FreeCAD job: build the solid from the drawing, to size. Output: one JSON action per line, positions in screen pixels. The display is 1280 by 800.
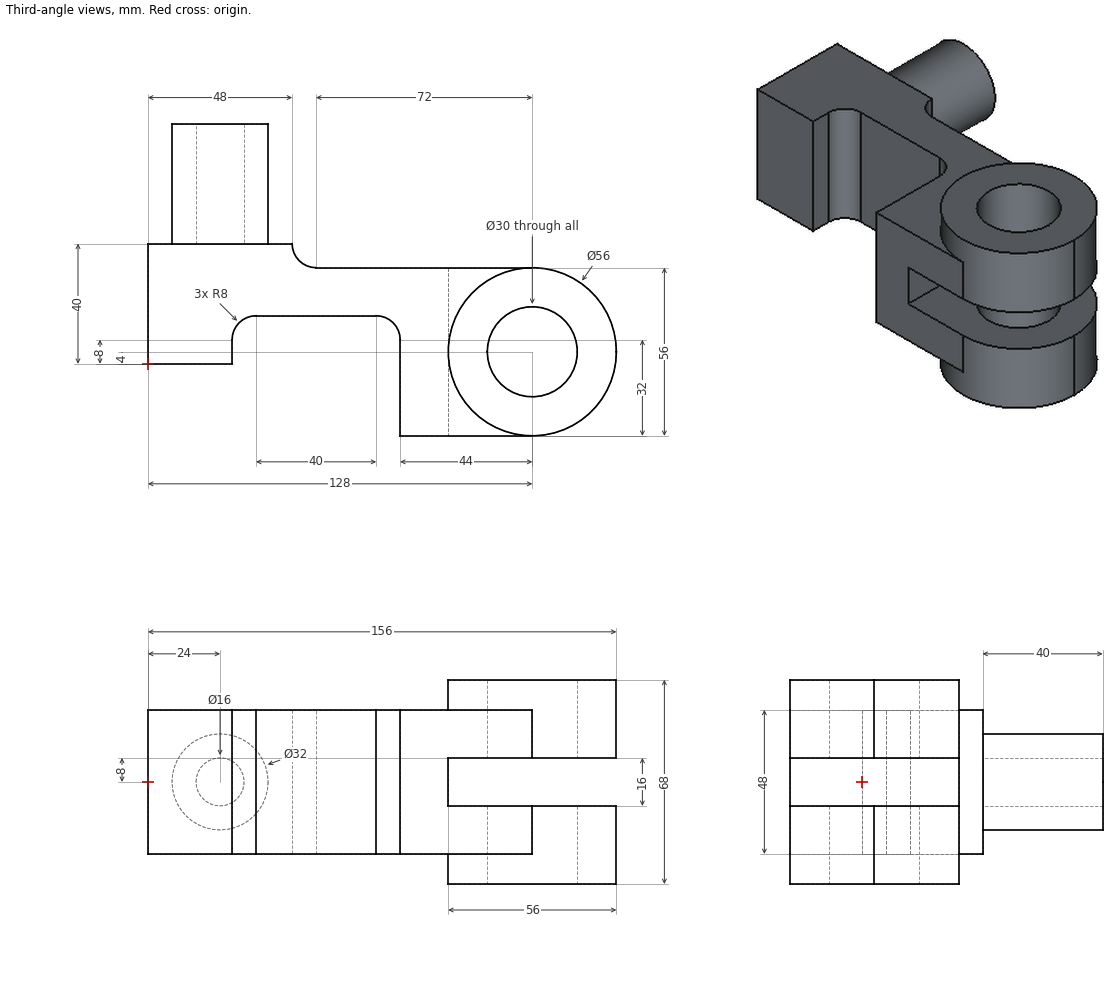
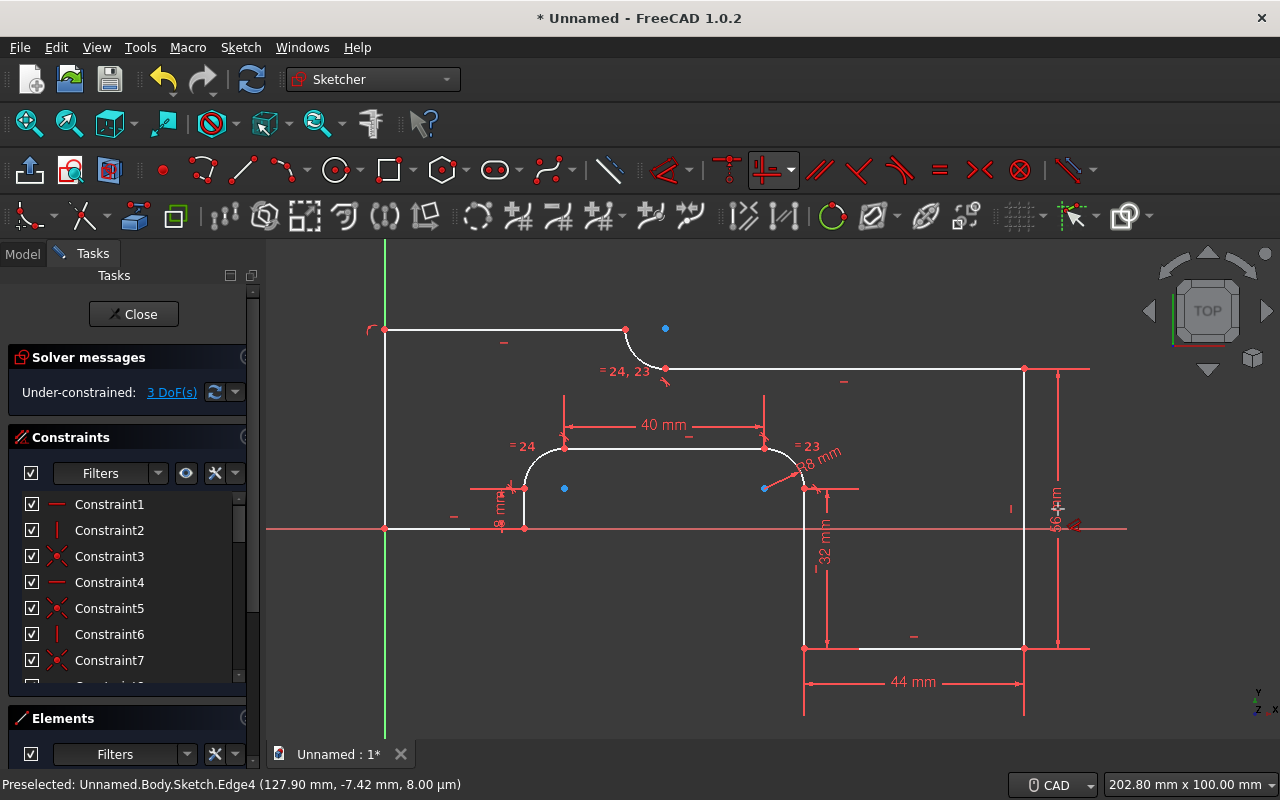
{"action": "left_click", "coordinate": [917, 369]}
{"action": "left_click", "coordinate": [845, 335]}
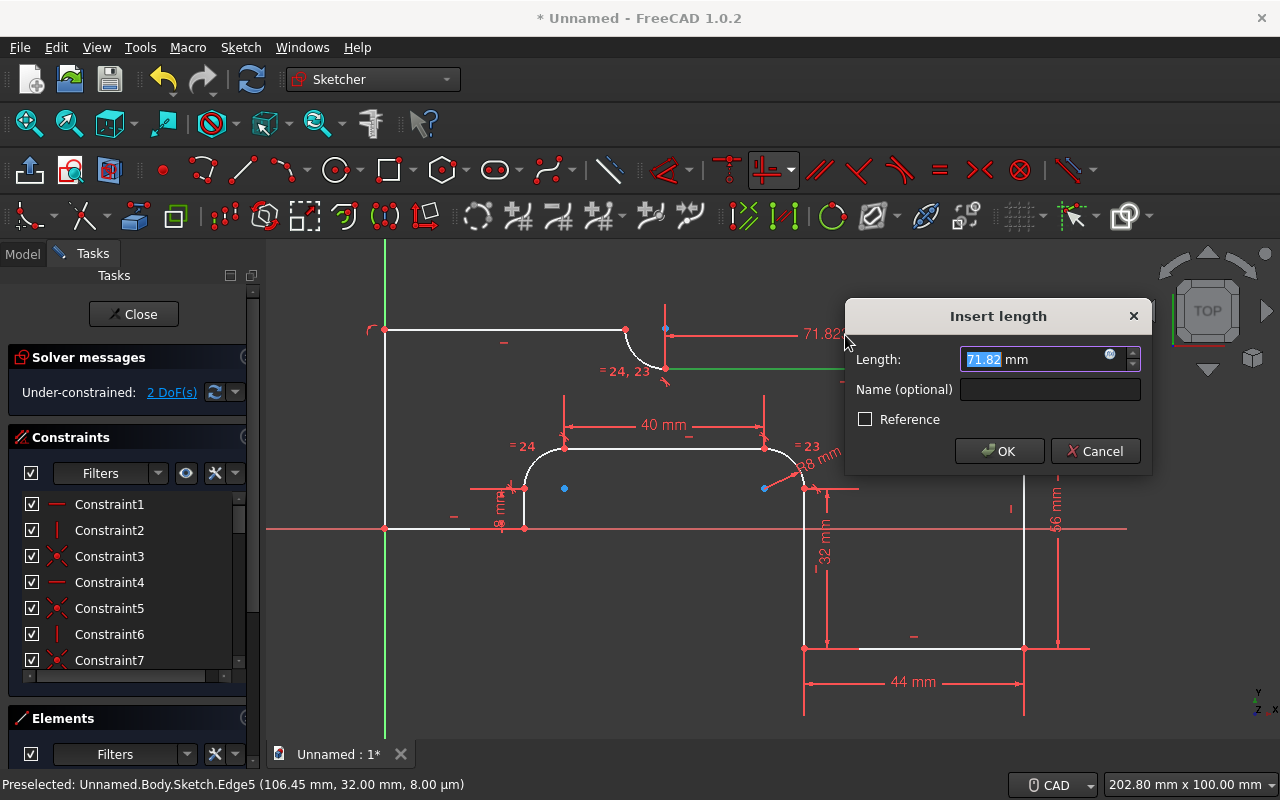
{"action": "type", "text": "72"}
{"action": "key", "text": "Return"}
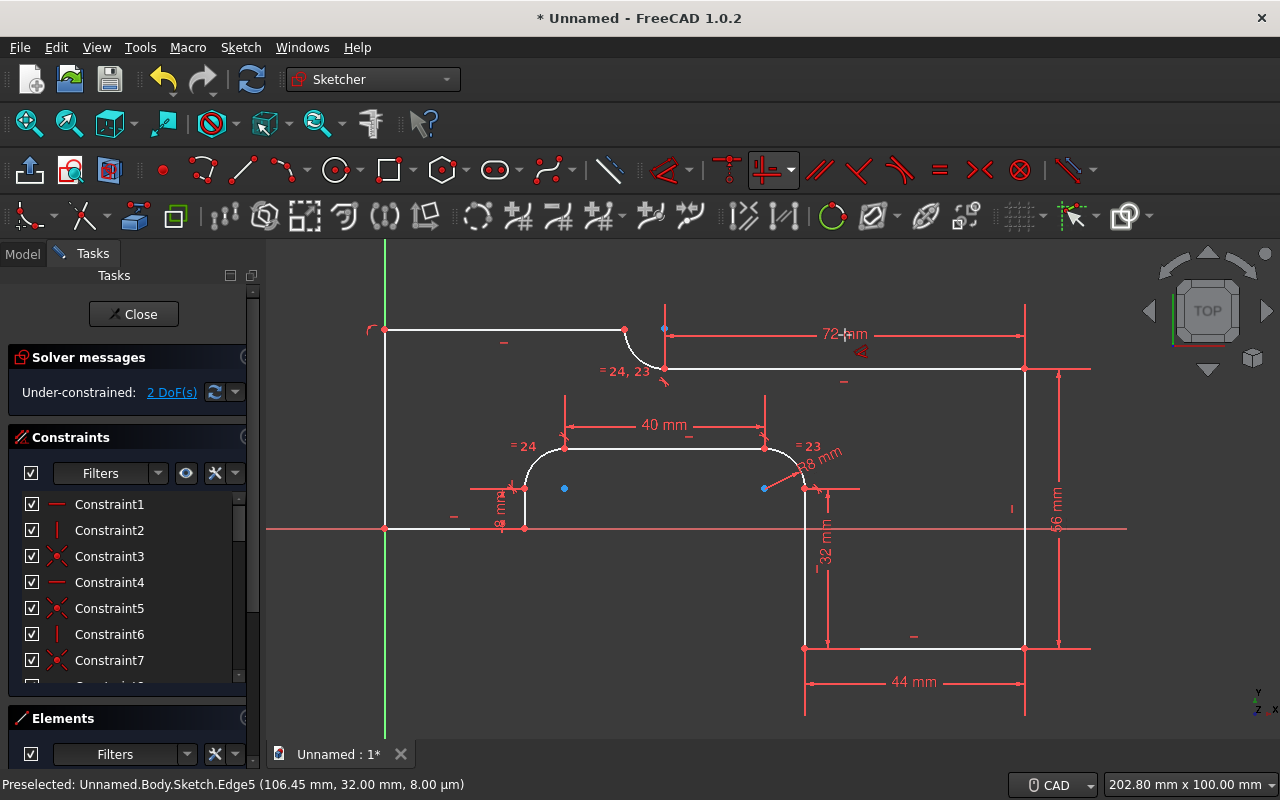
{"action": "left_click", "coordinate": [553, 330]}
{"action": "left_click", "coordinate": [505, 296]}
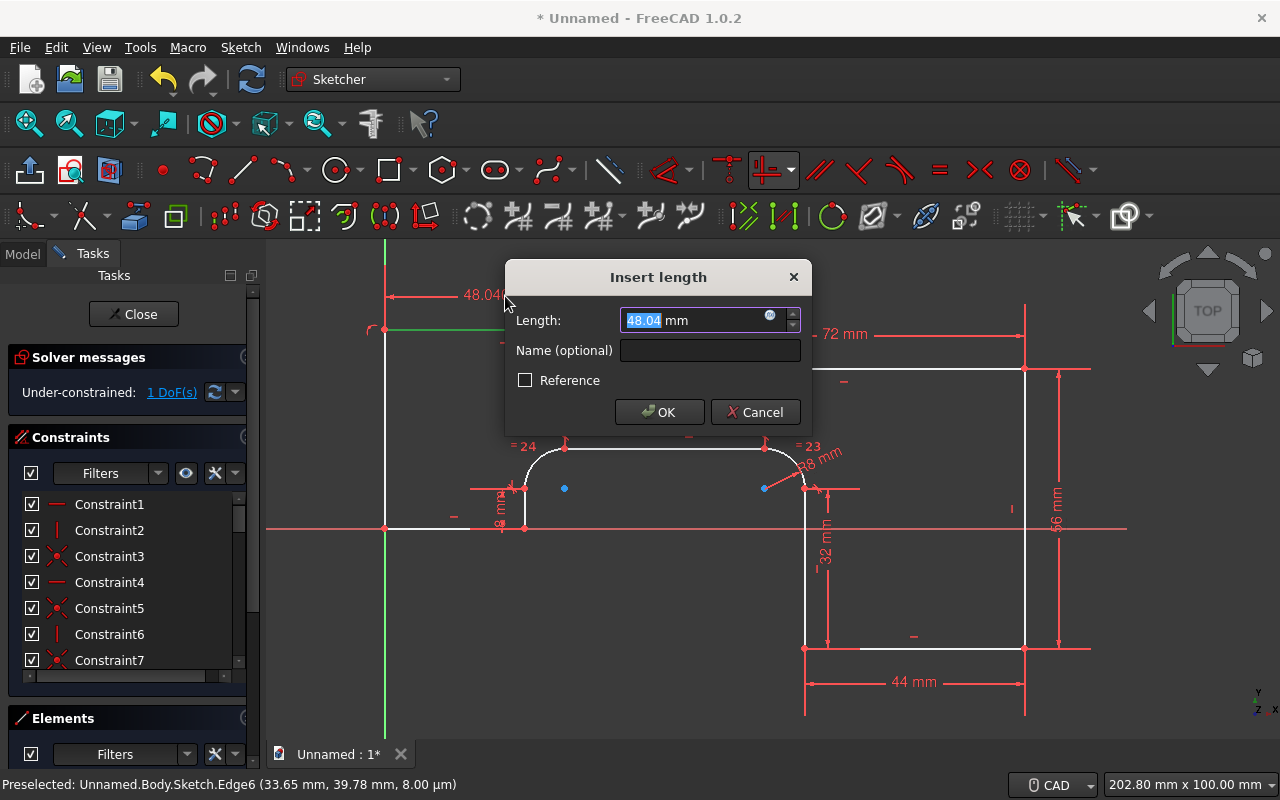
{"action": "type", "text": "48"}
{"action": "key", "text": "Return"}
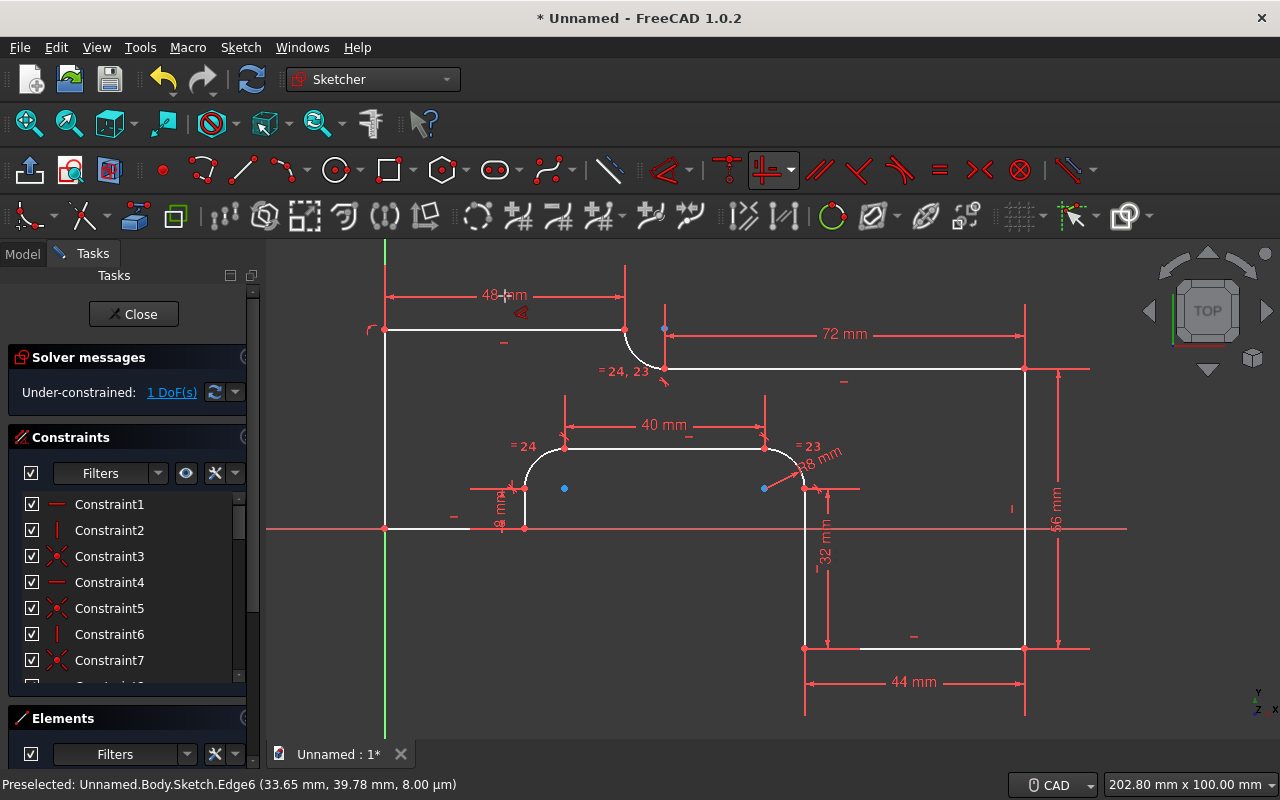
{"action": "left_click", "coordinate": [385, 390]}
{"action": "left_click", "coordinate": [351, 429]}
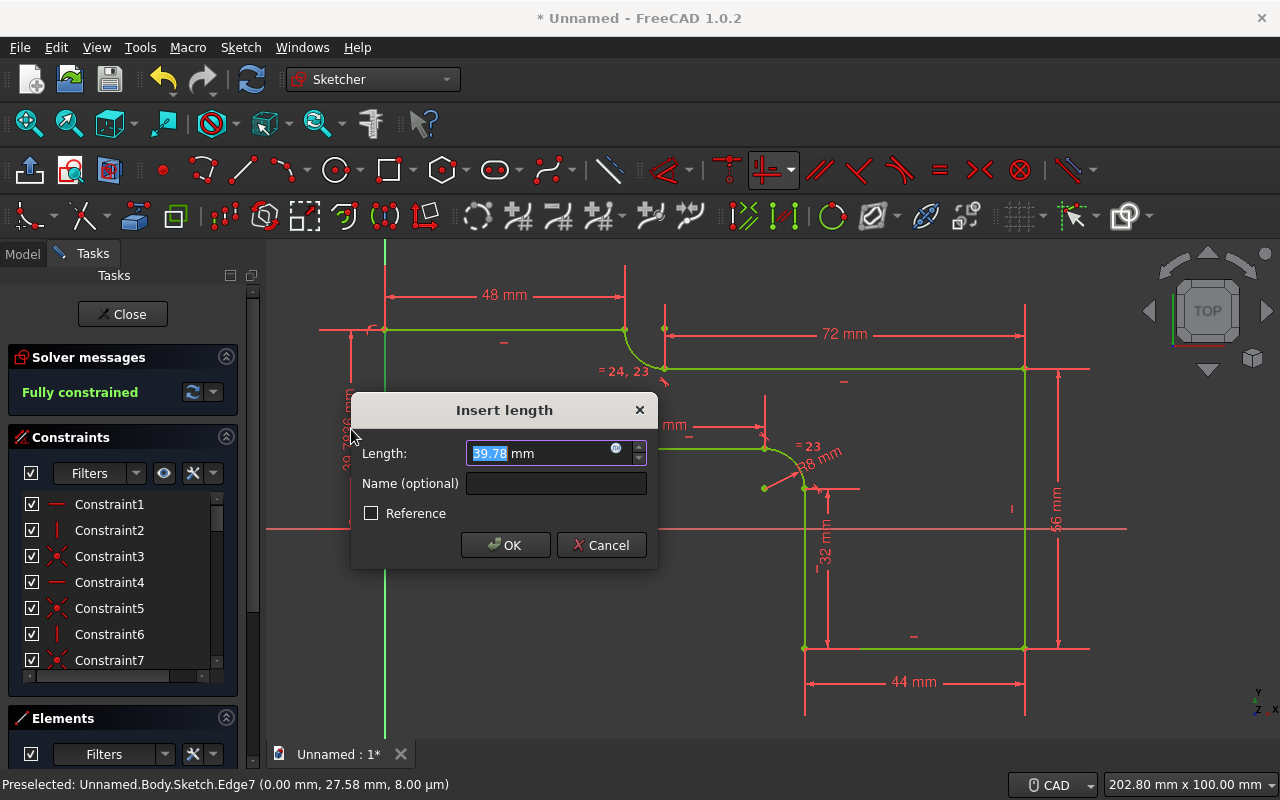
{"action": "type", "text": "40"}
{"action": "key", "text": "Return"}
{"action": "key", "text": "Escape"}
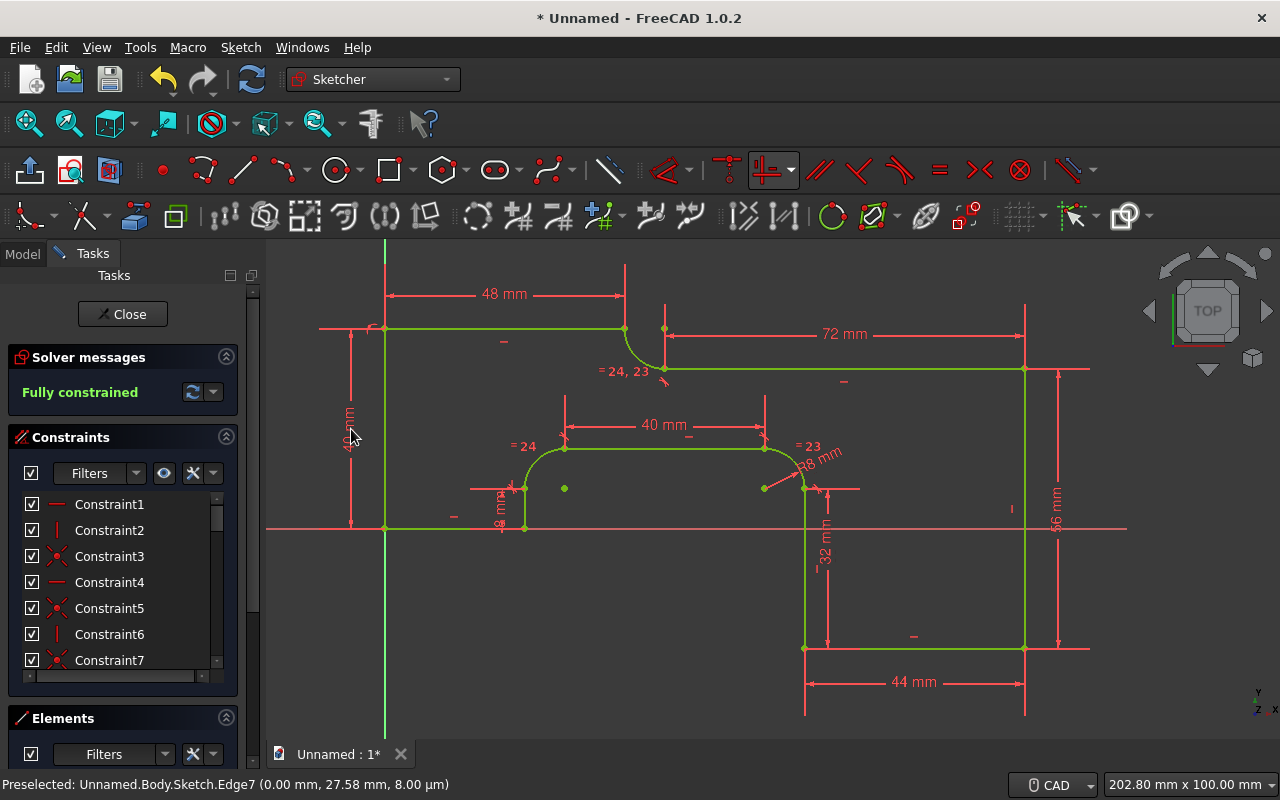
{"action": "left_click", "coordinate": [123, 314]}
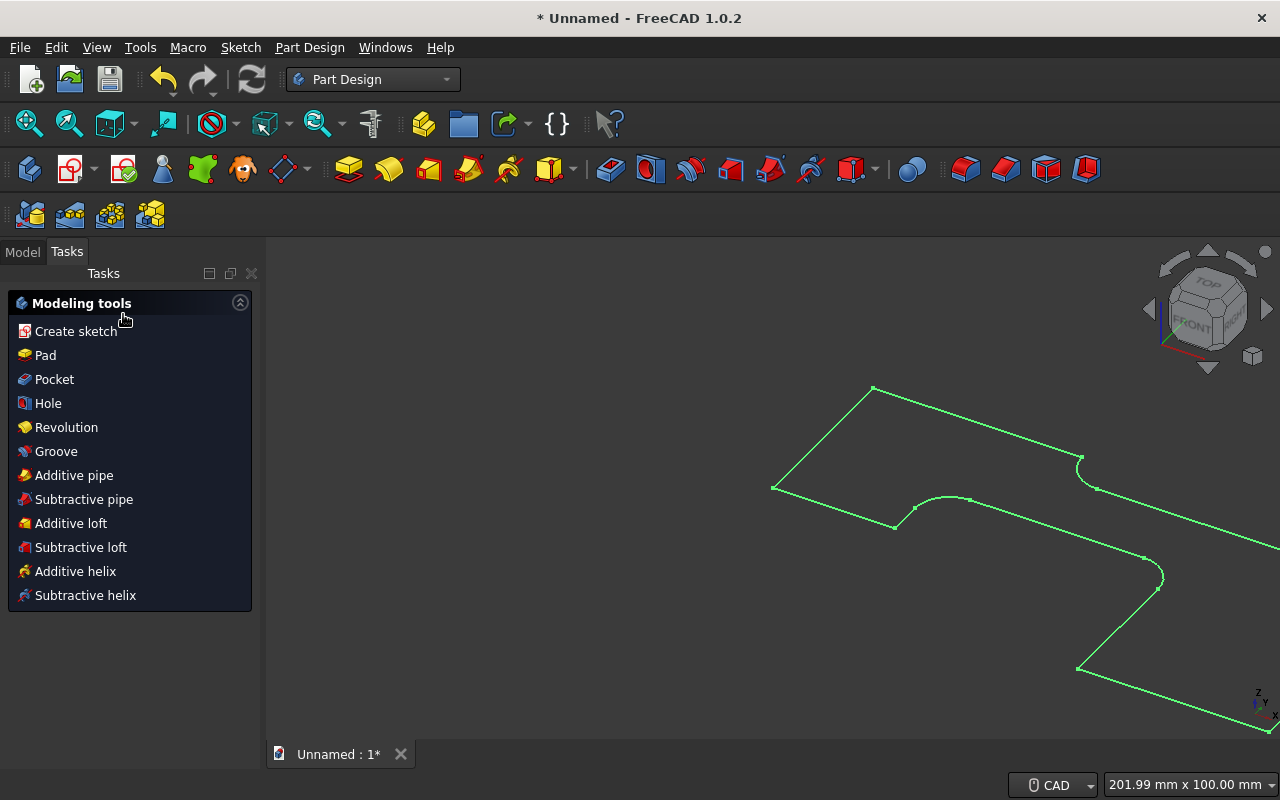
{"action": "left_click", "coordinate": [350, 170]}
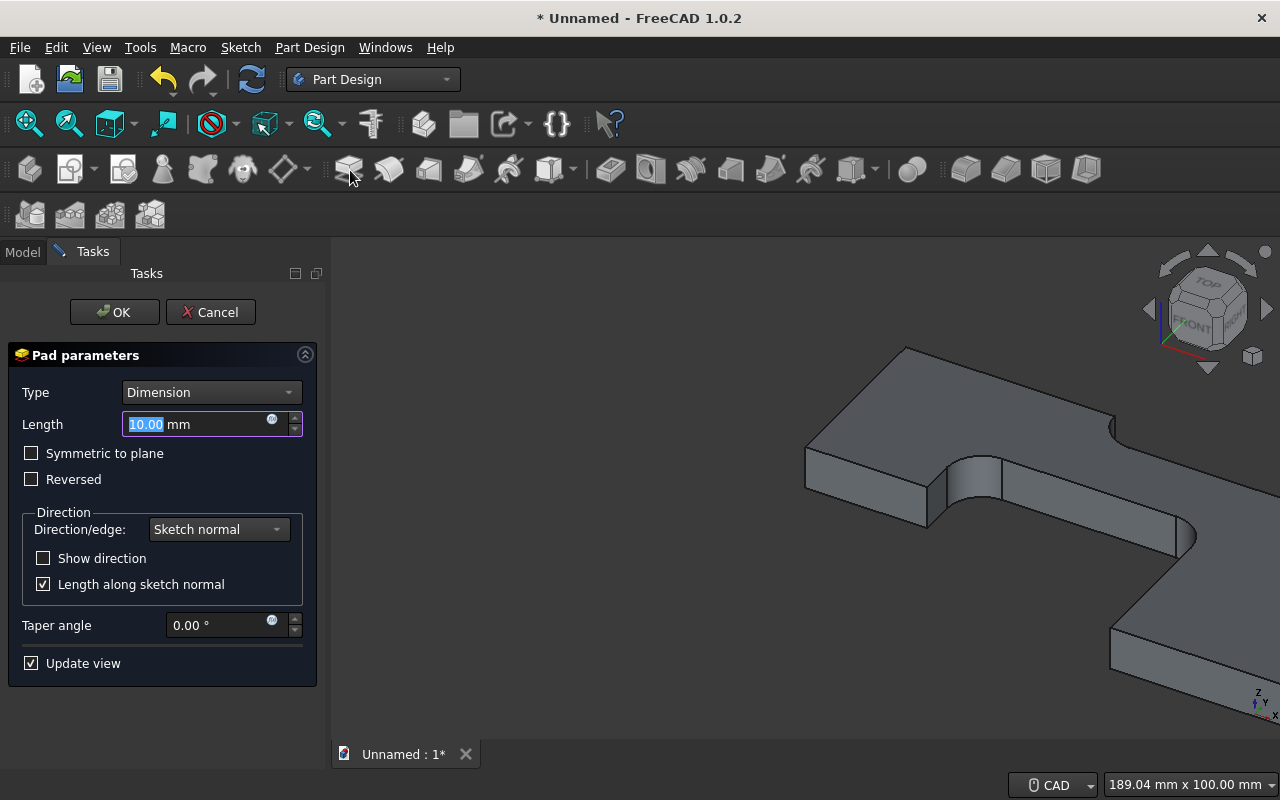
{"action": "type", "text": "48"}
{"action": "key", "text": "Tab"}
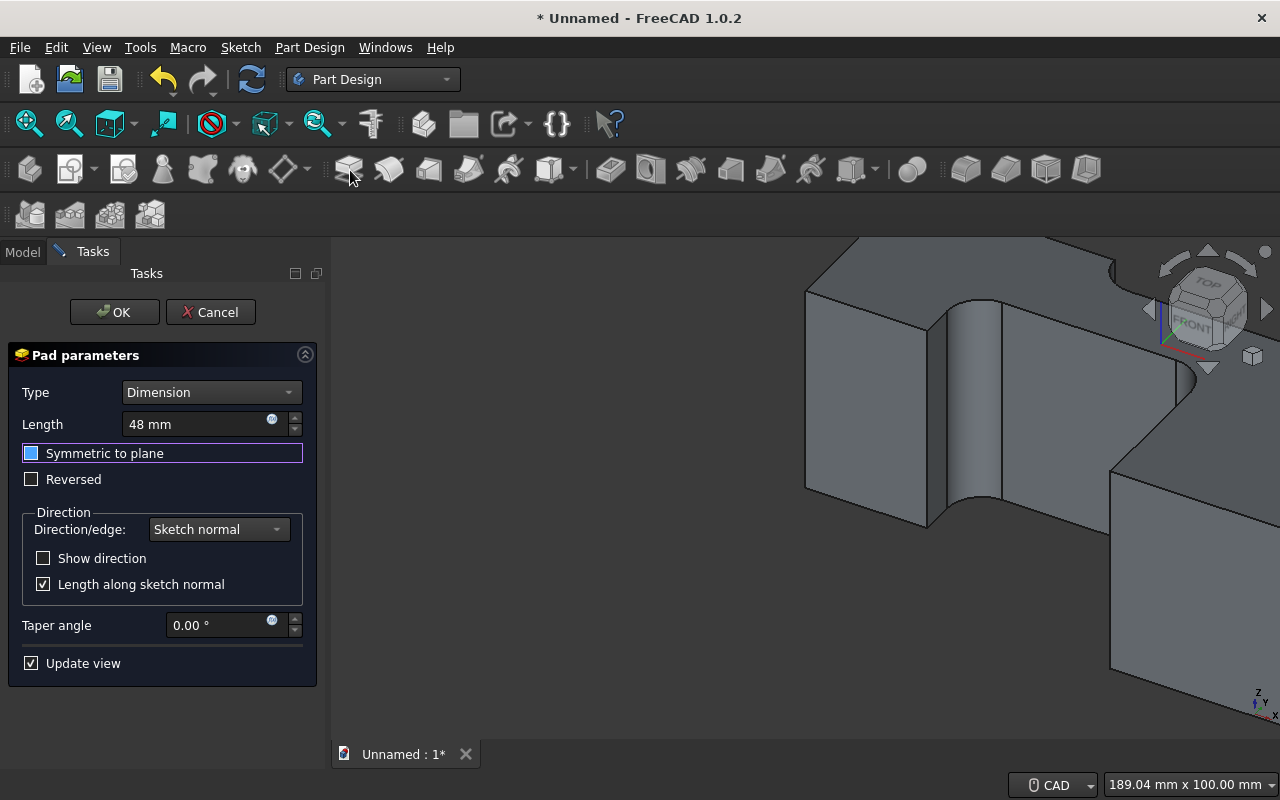
{"action": "left_click", "coordinate": [30, 453]}